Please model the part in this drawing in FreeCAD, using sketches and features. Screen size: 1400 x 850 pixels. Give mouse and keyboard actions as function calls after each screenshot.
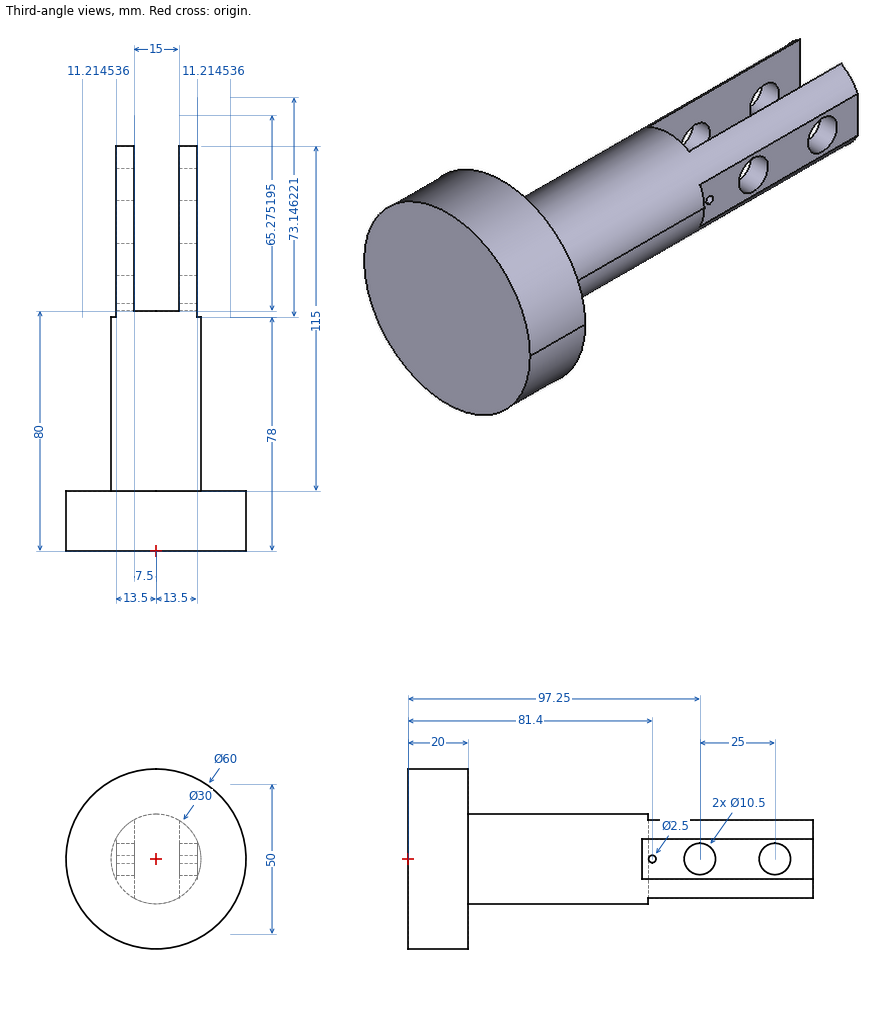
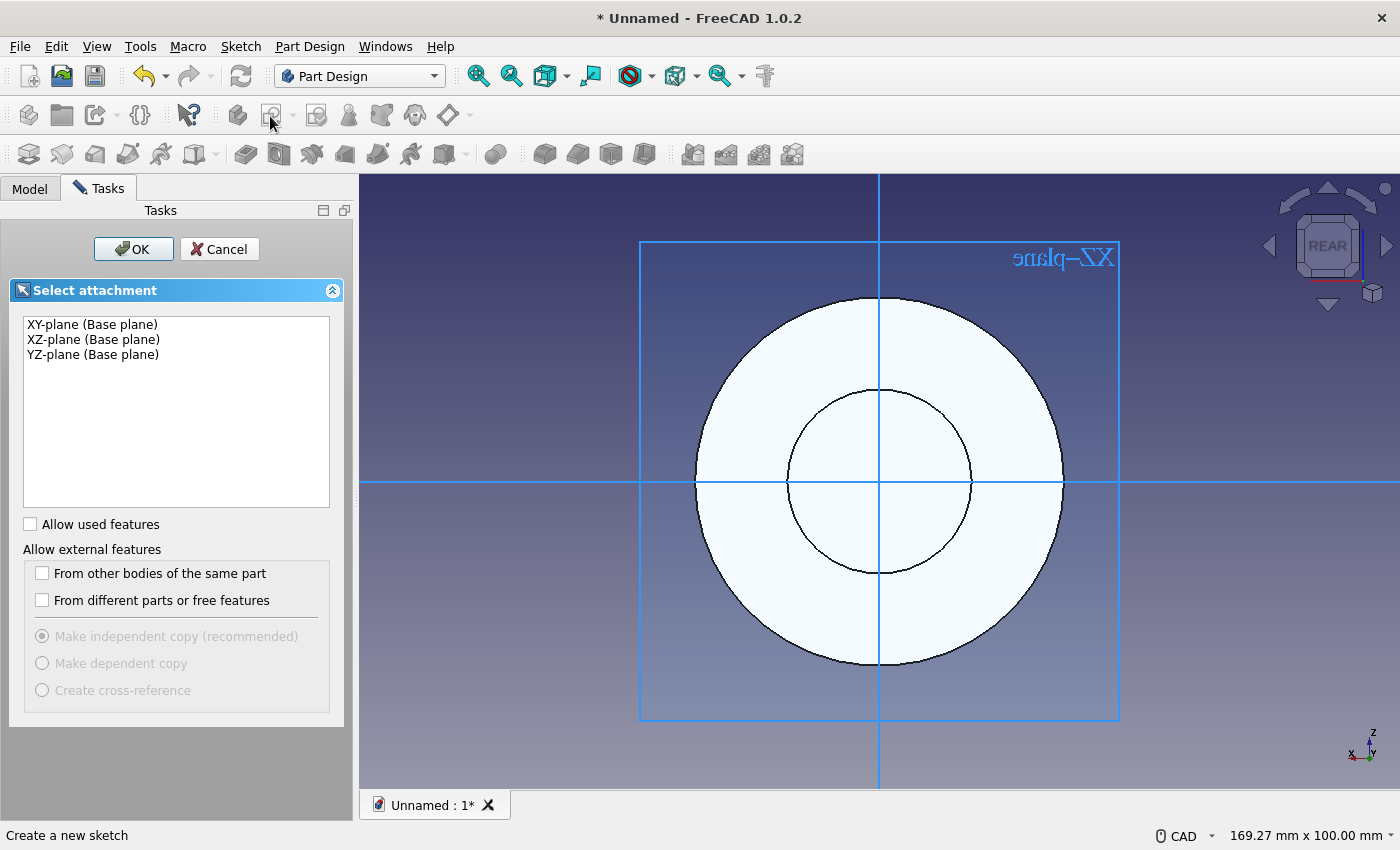
click(84, 324)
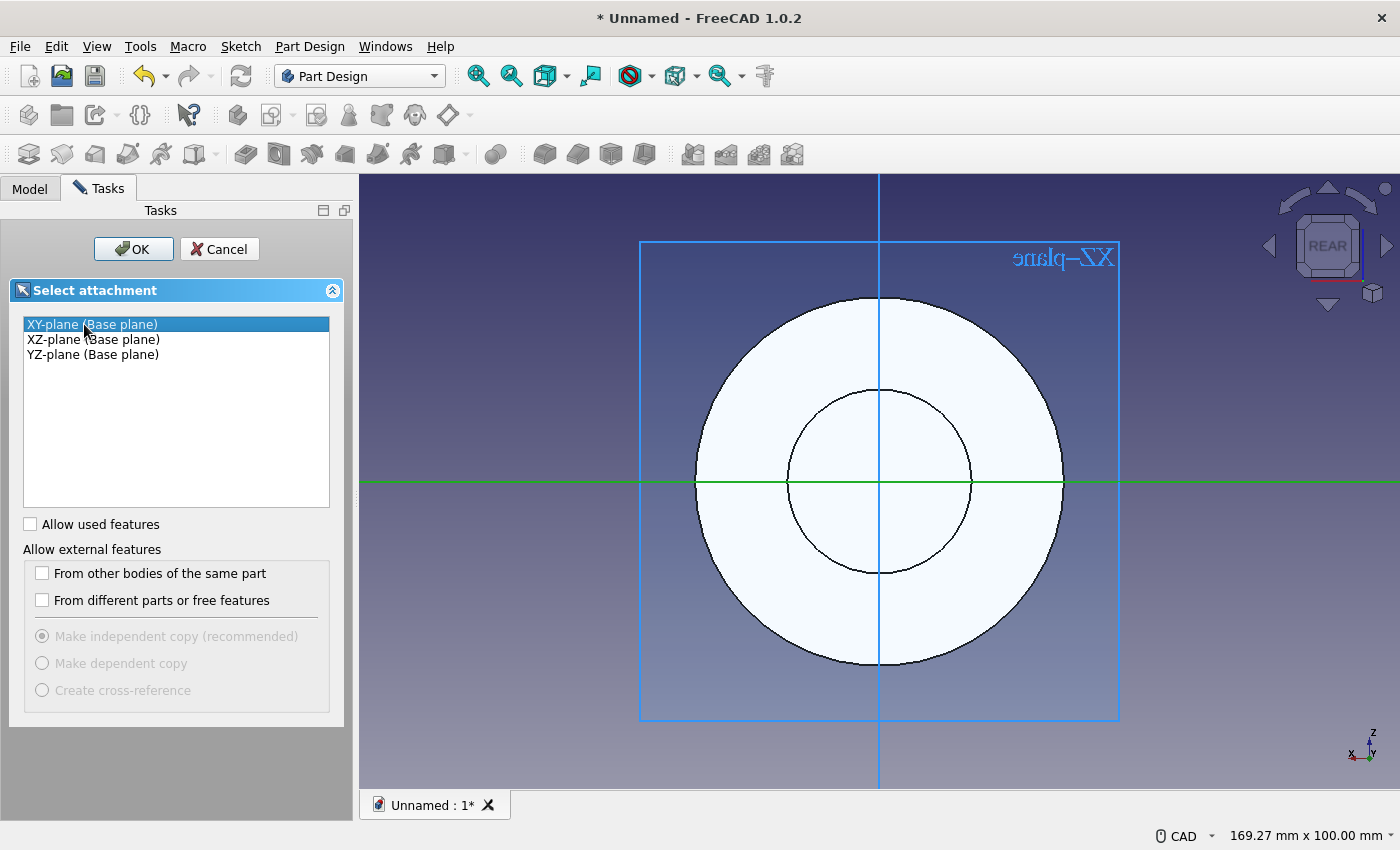
click(134, 249)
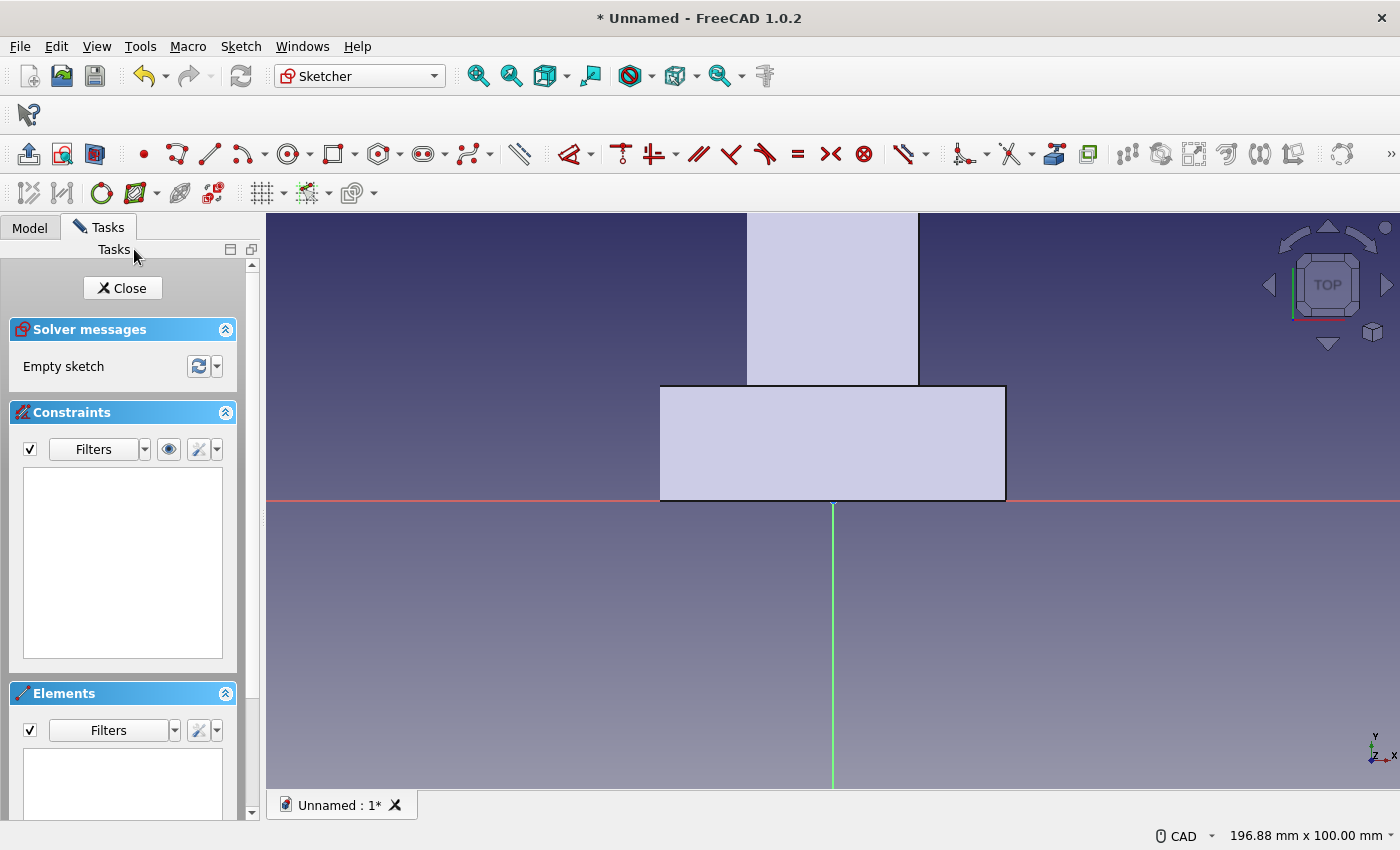
click(95, 154)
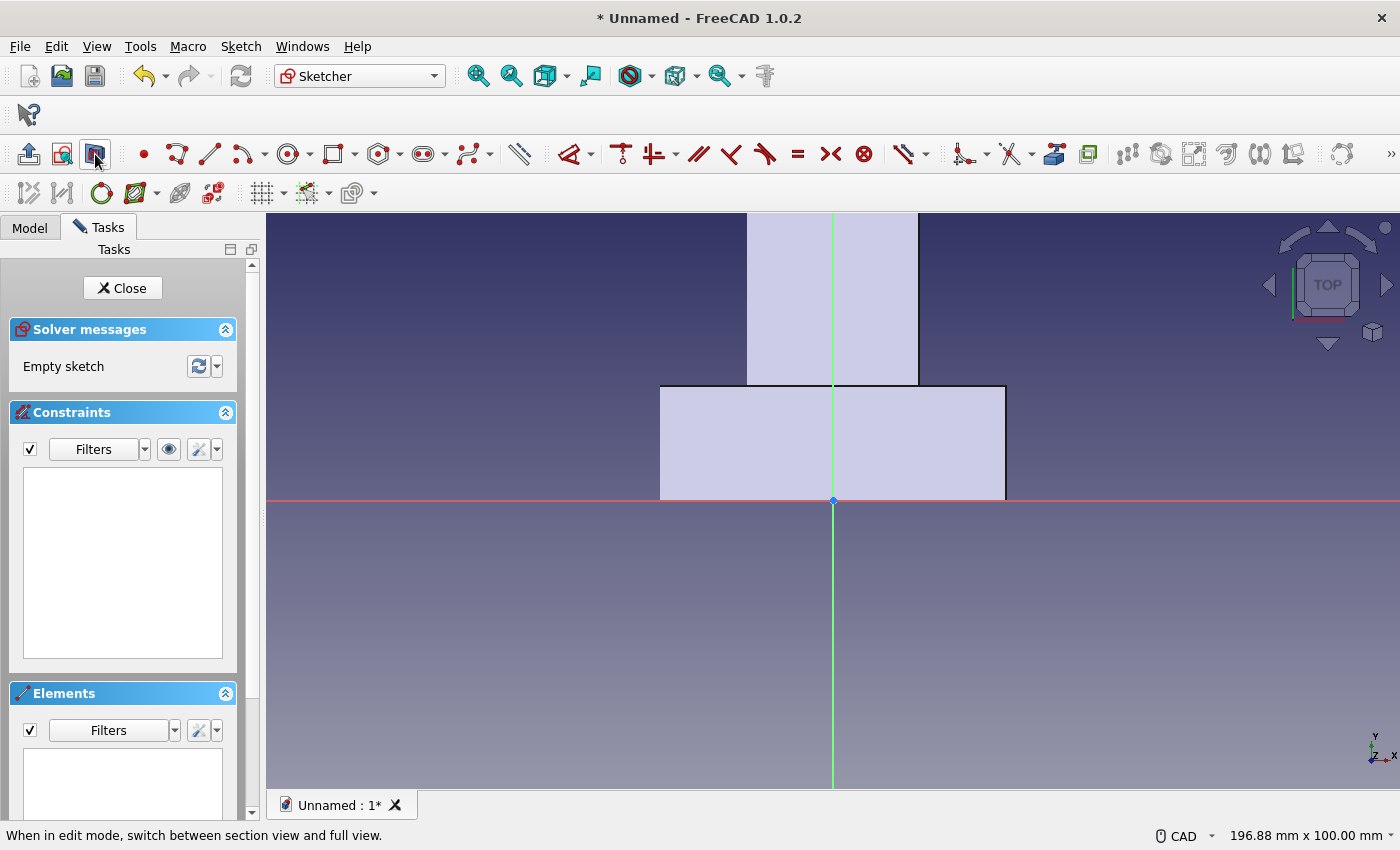
scroll(709, 761, down, 4)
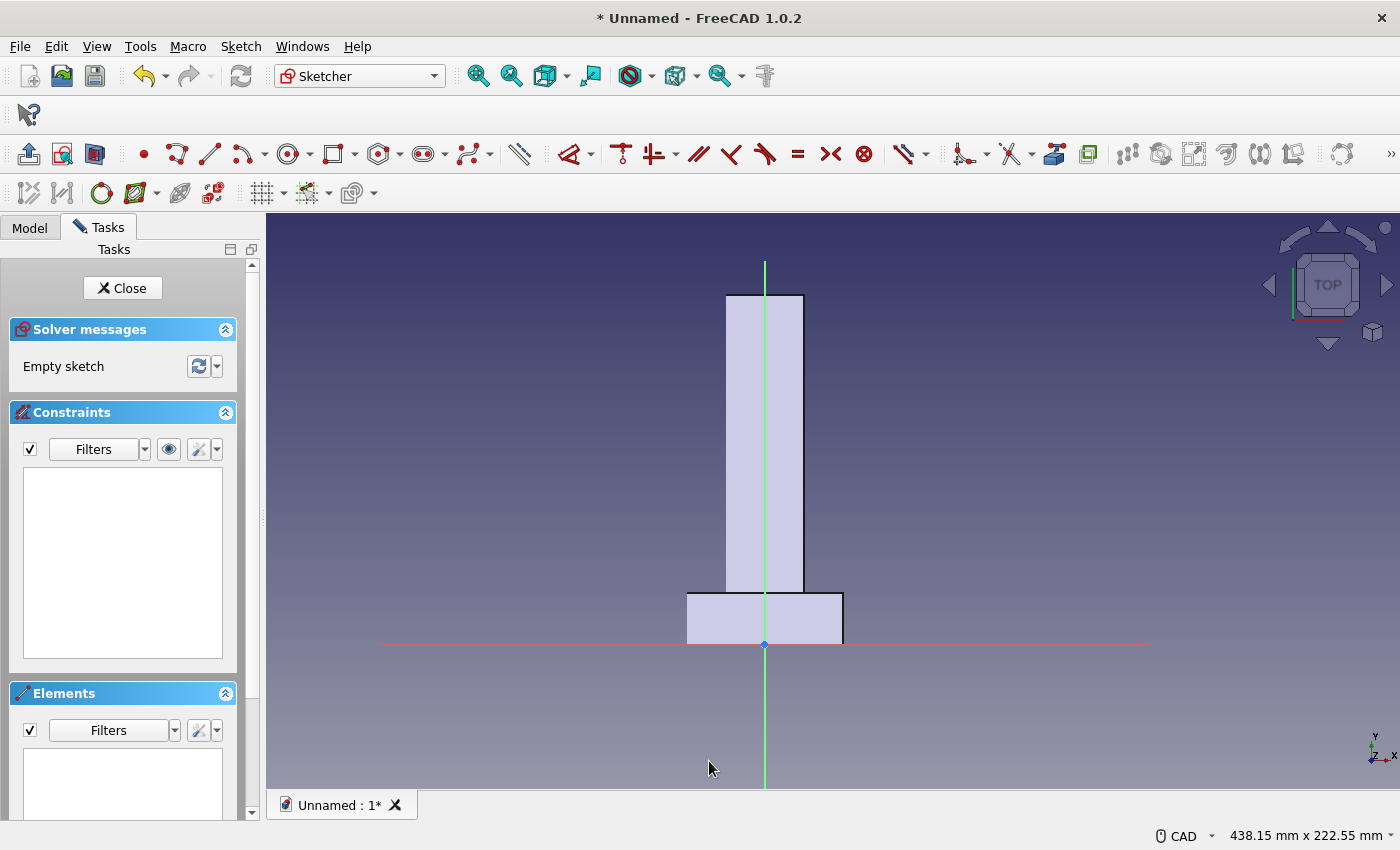
click(332, 154)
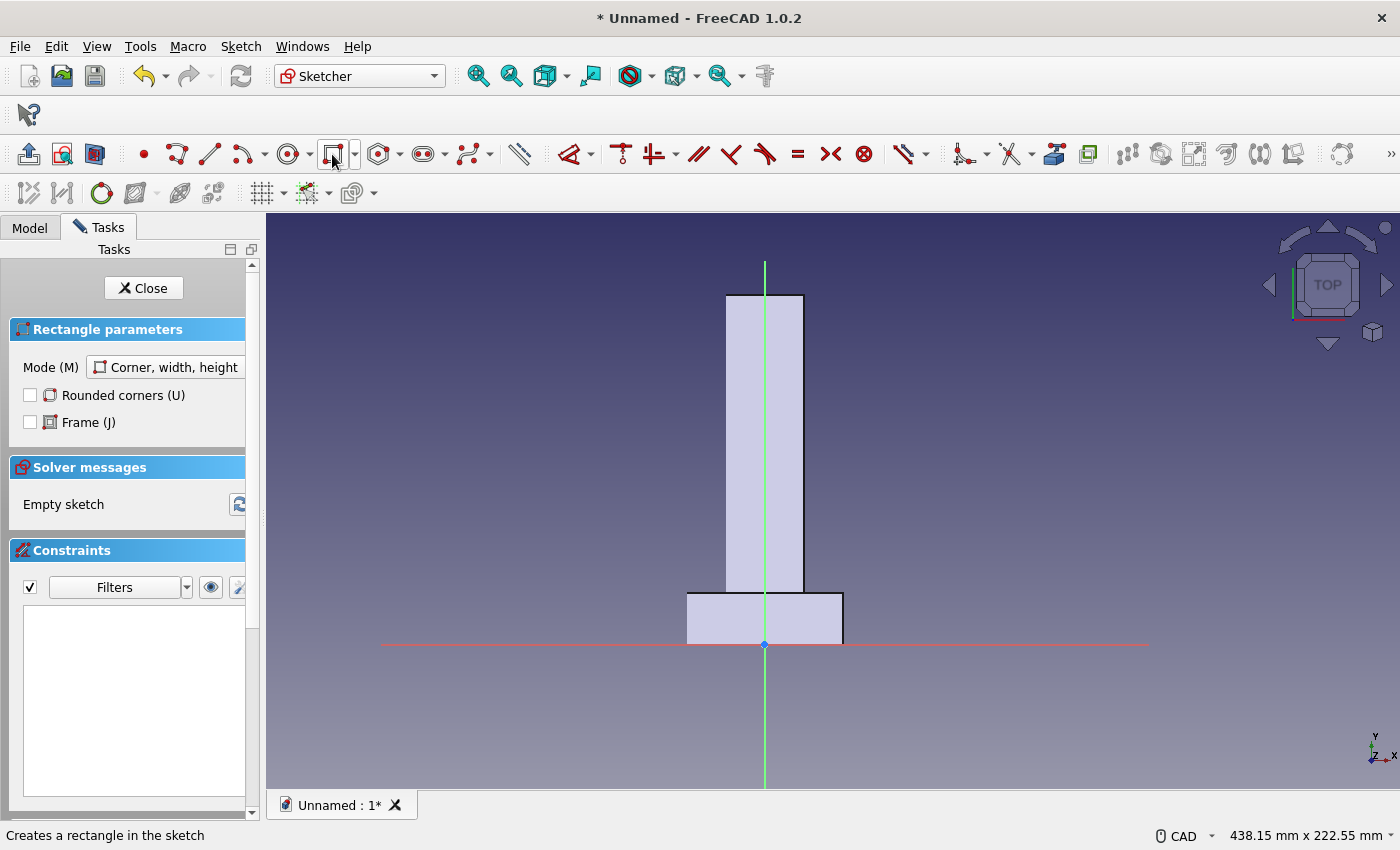
click(746, 269)
move(784, 438)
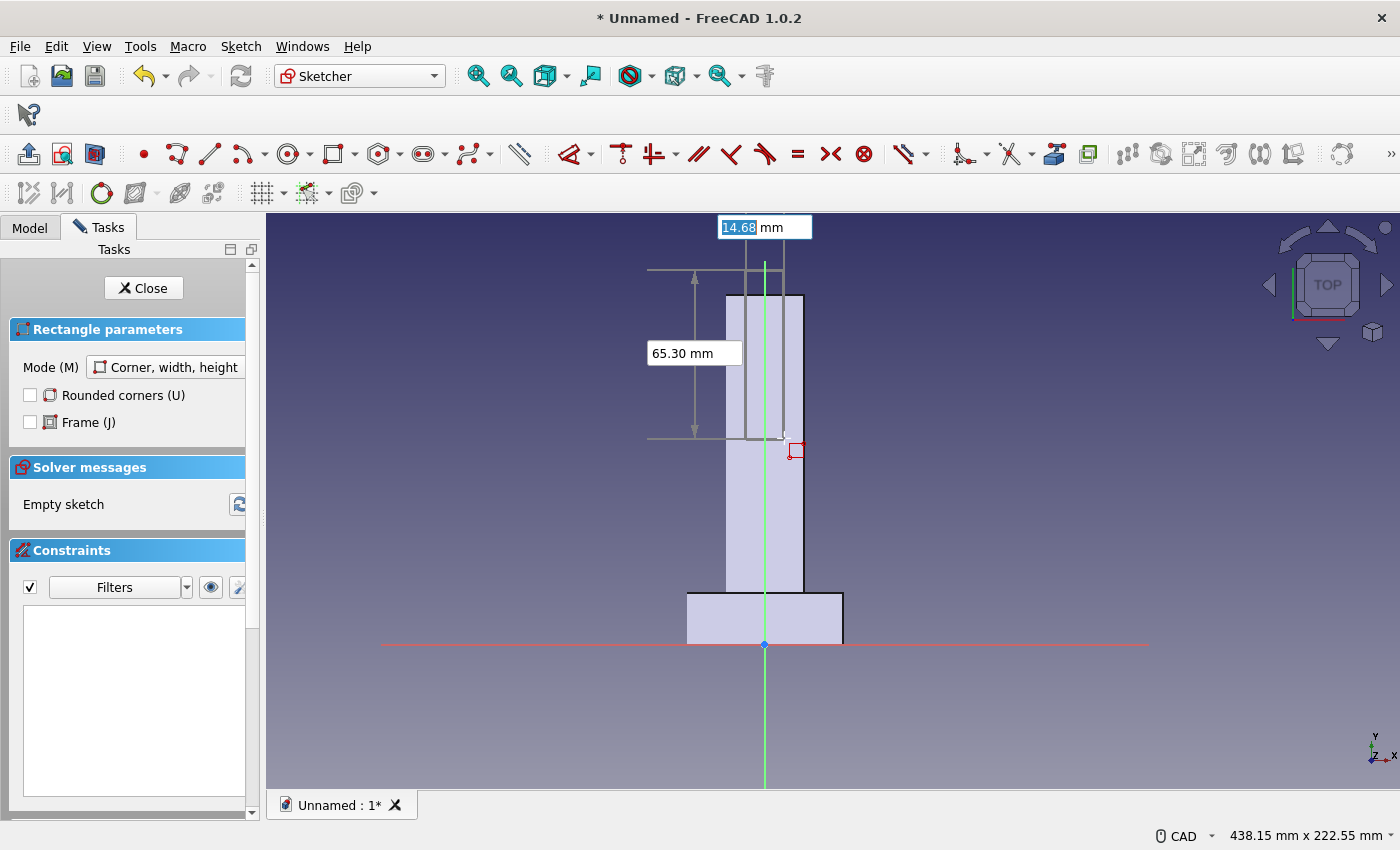
text(15)
key(Tab)
text(65.275195)
key(Return)
key(Escape)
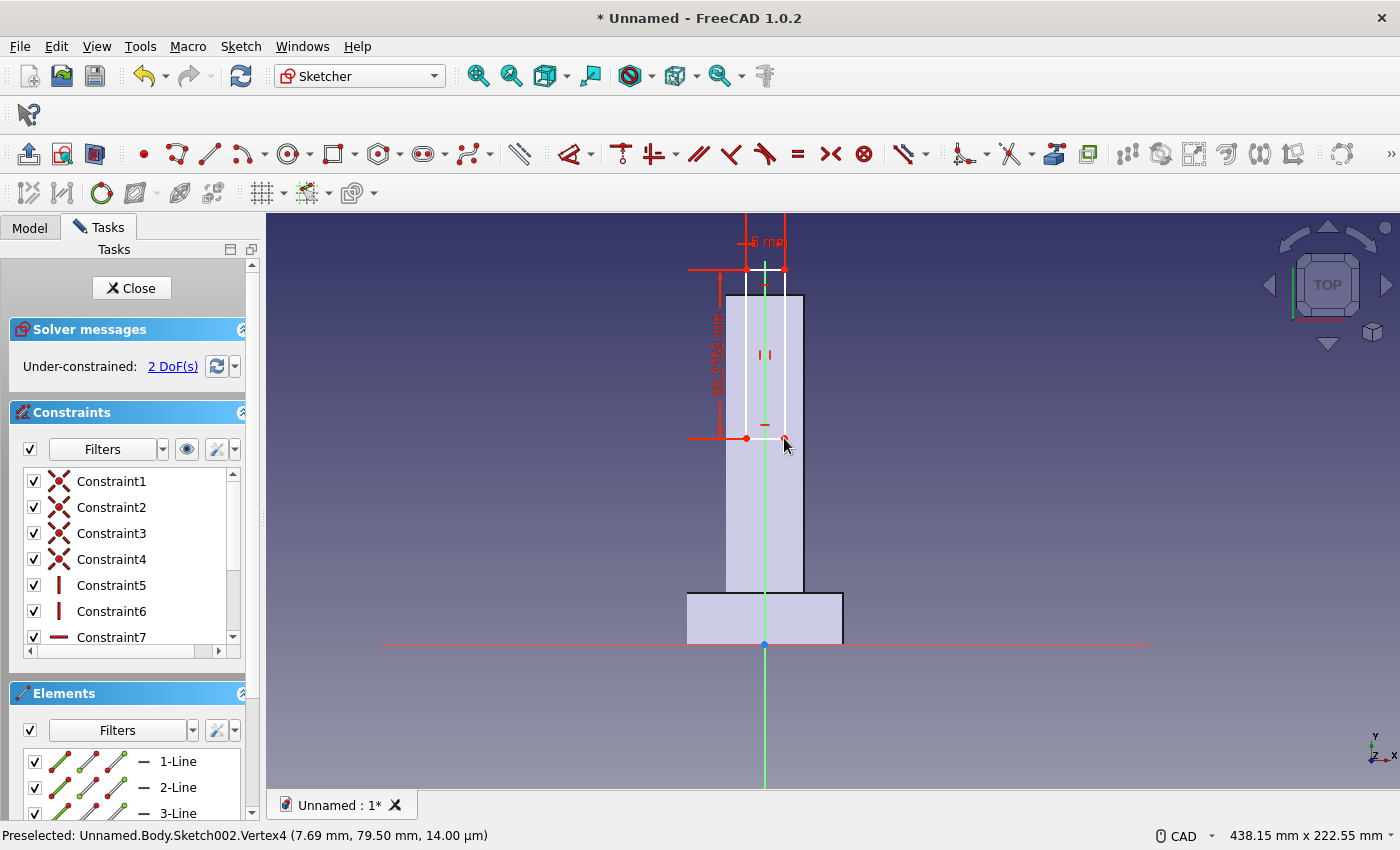
click(568, 154)